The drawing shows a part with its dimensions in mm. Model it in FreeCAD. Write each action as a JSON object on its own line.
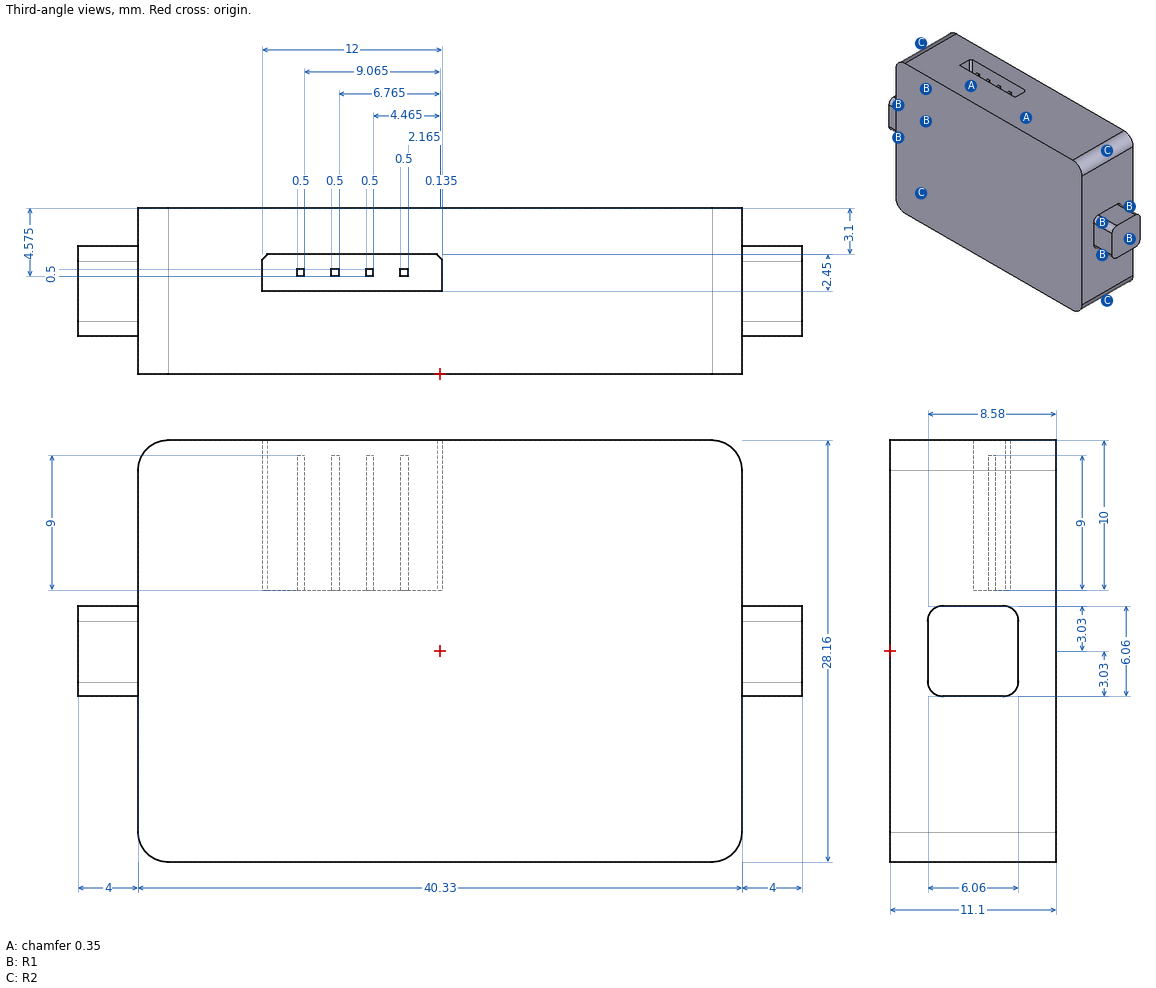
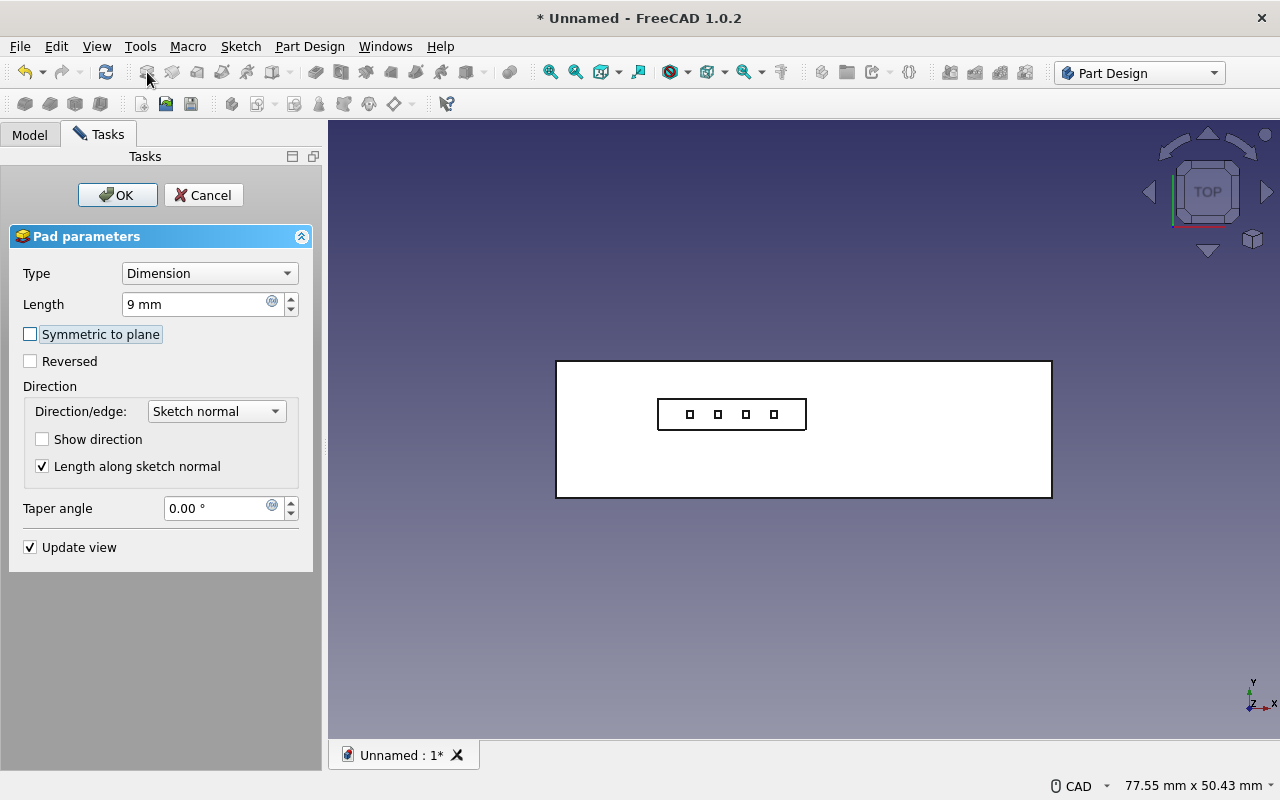
{"action": "left_click", "coordinate": [118, 195]}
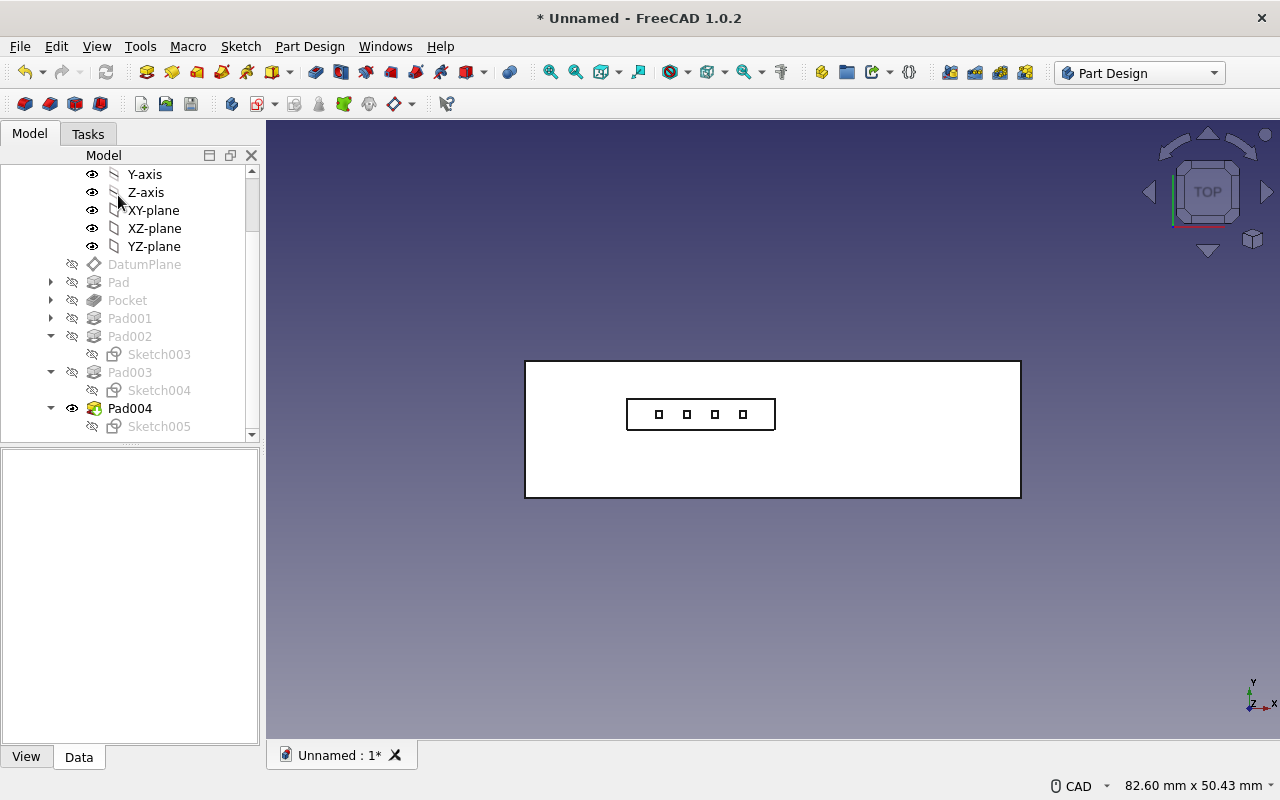
{"action": "key", "text": "6"}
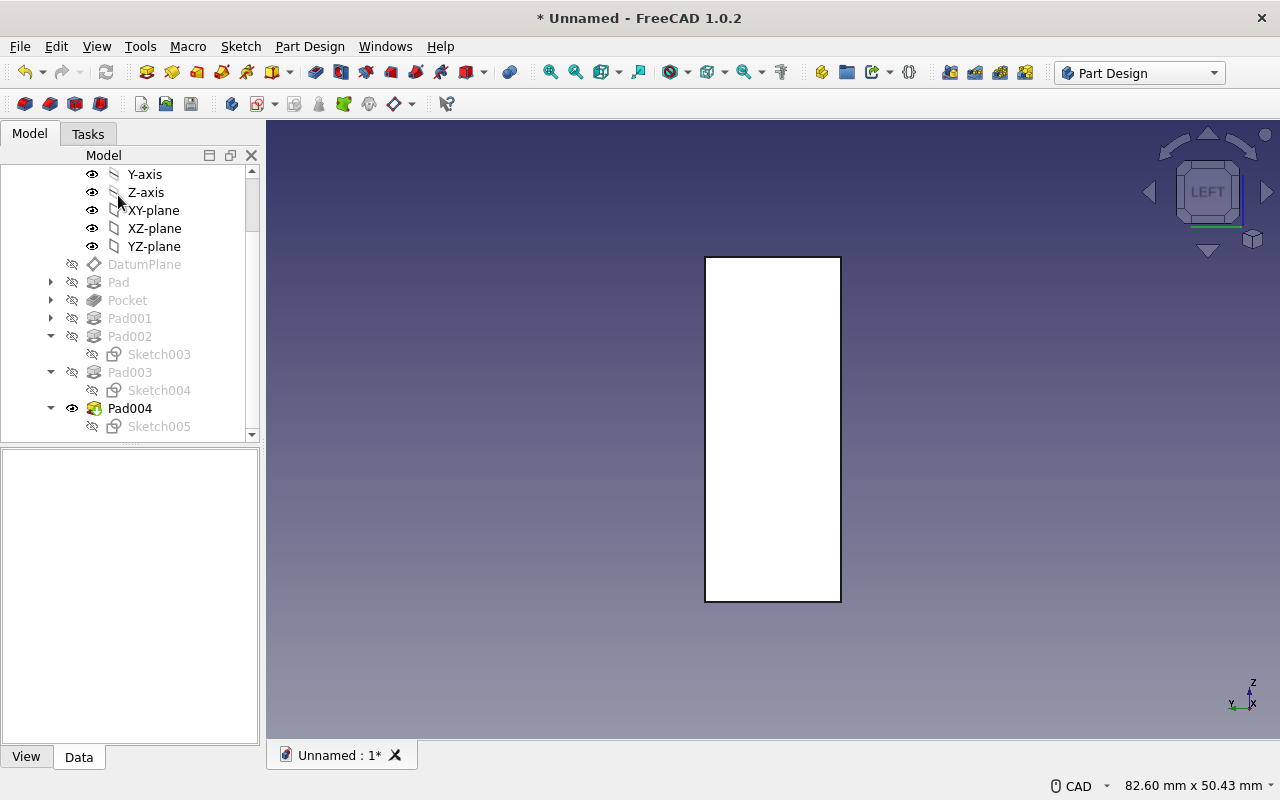
{"action": "left_click", "coordinate": [773, 330]}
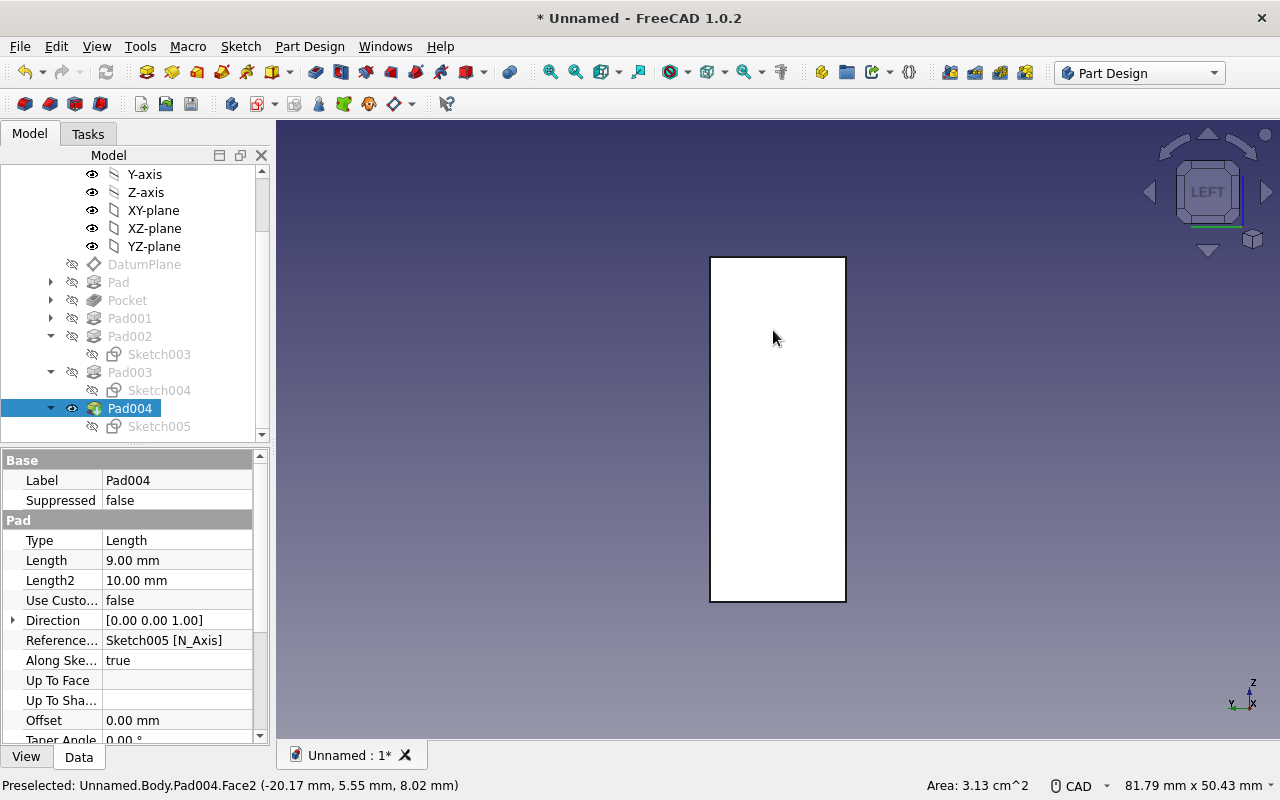
{"action": "left_click", "coordinate": [256, 104]}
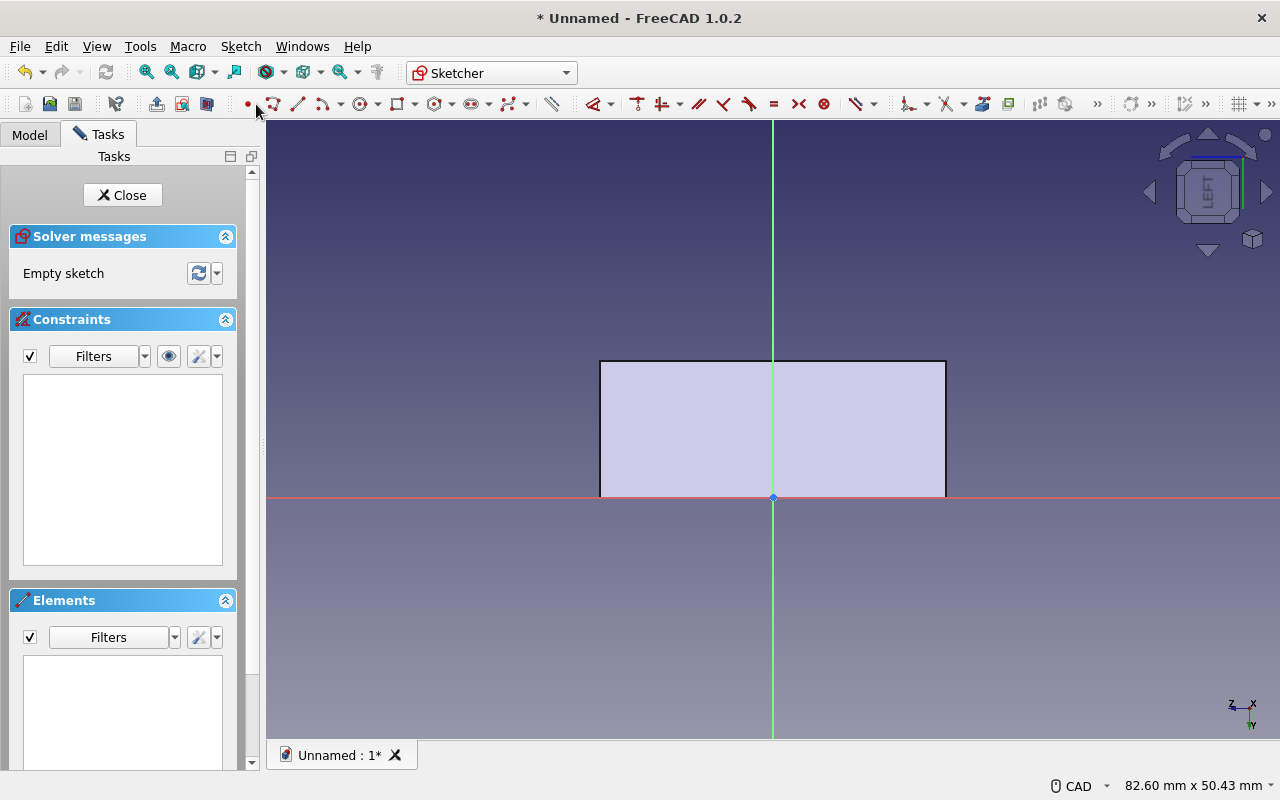
{"action": "scroll", "coordinate": [795, 450], "scroll_direction": "up", "scroll_amount": 7}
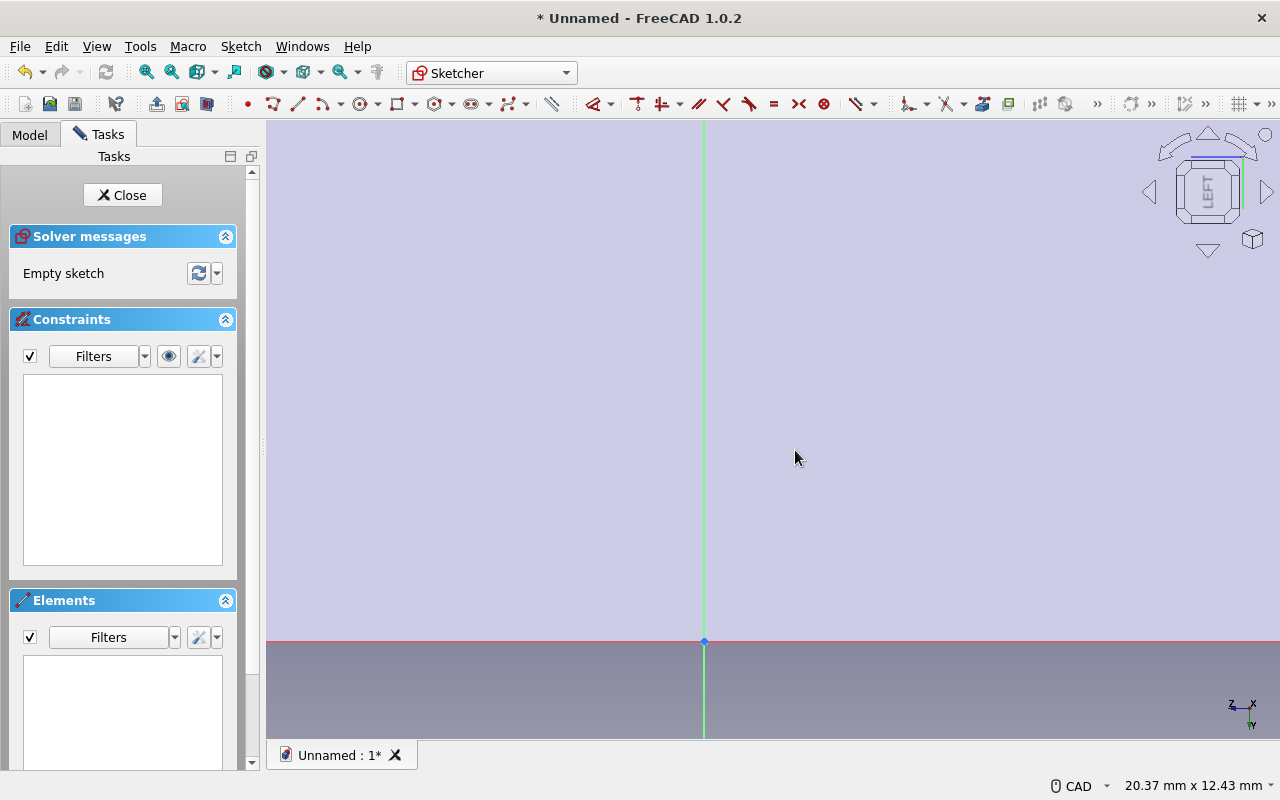
{"action": "left_click", "coordinate": [396, 104]}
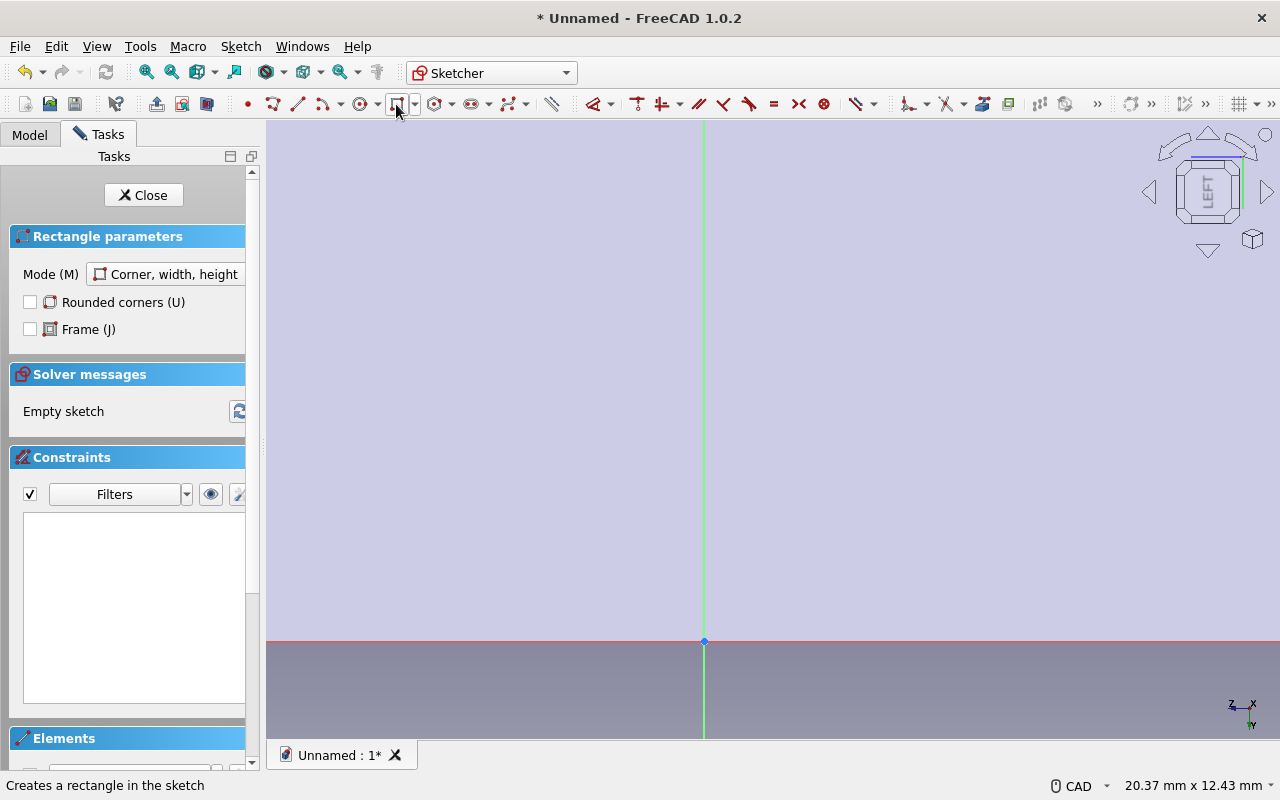
{"action": "left_click", "coordinate": [553, 214]}
{"action": "mouse_move", "coordinate": [855, 516]}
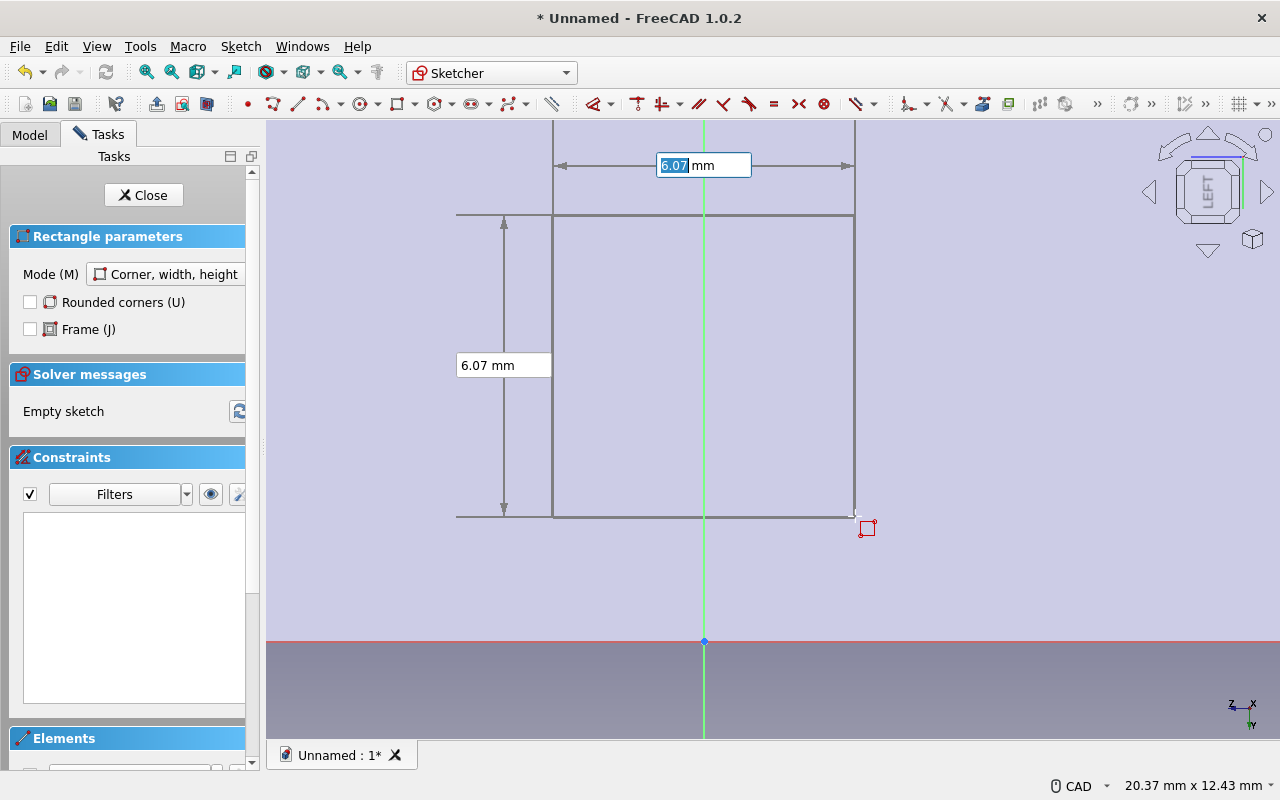
{"action": "type", "text": "6.06"}
{"action": "key", "text": "Tab"}
{"action": "type", "text": "6.06"}
{"action": "key", "text": "Return"}
{"action": "key", "text": "Escape"}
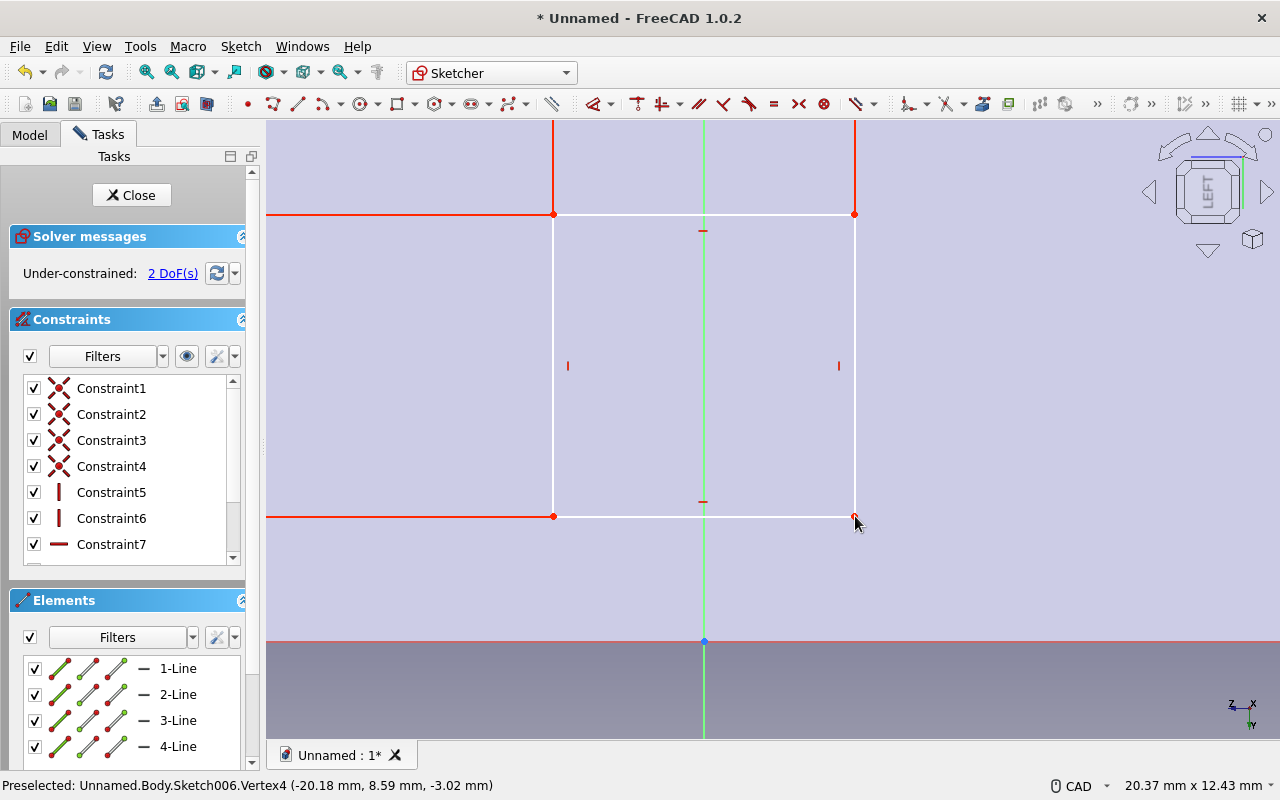
{"action": "left_click", "coordinate": [592, 104]}